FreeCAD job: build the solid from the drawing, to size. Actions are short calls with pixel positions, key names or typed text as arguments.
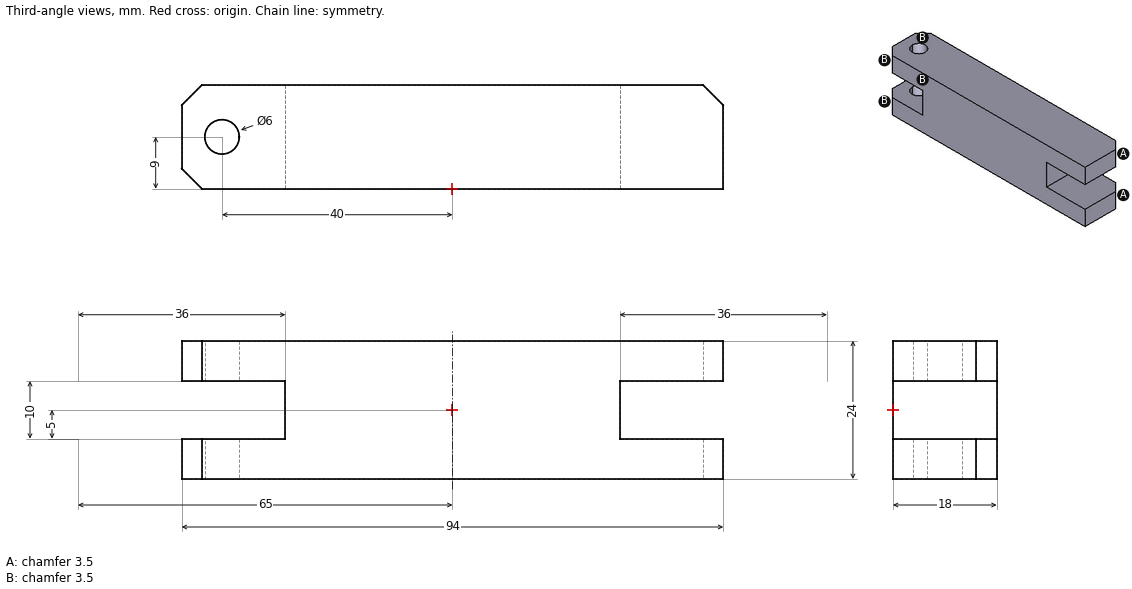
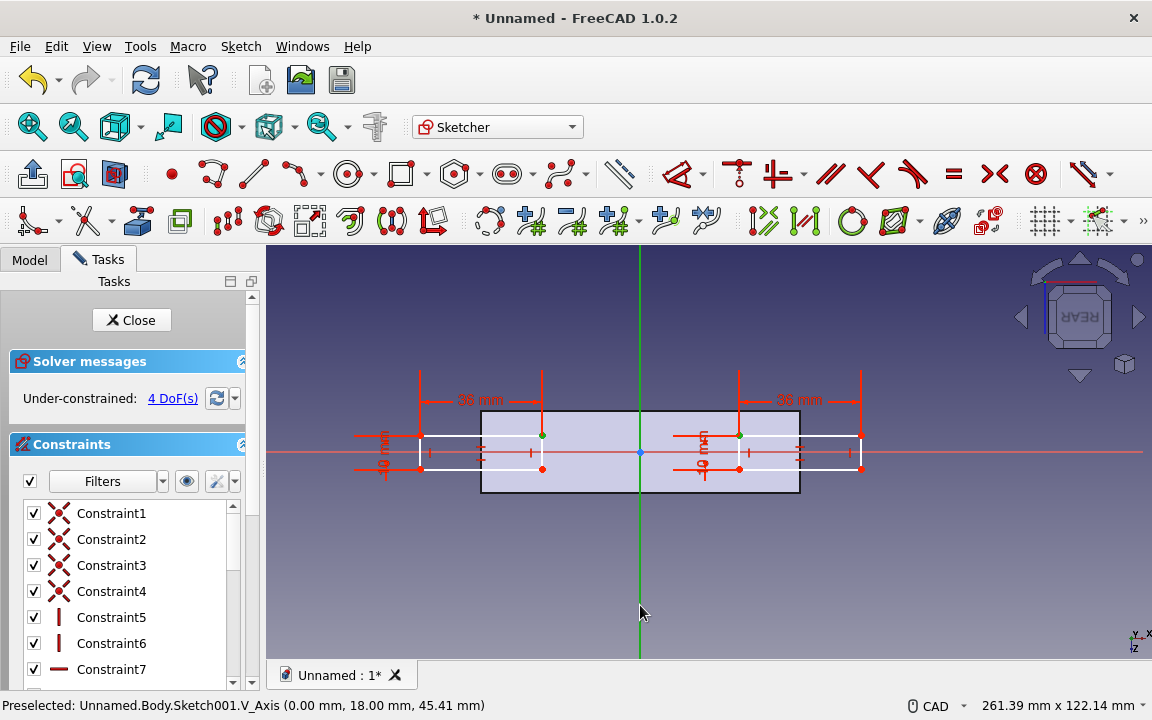
key(s)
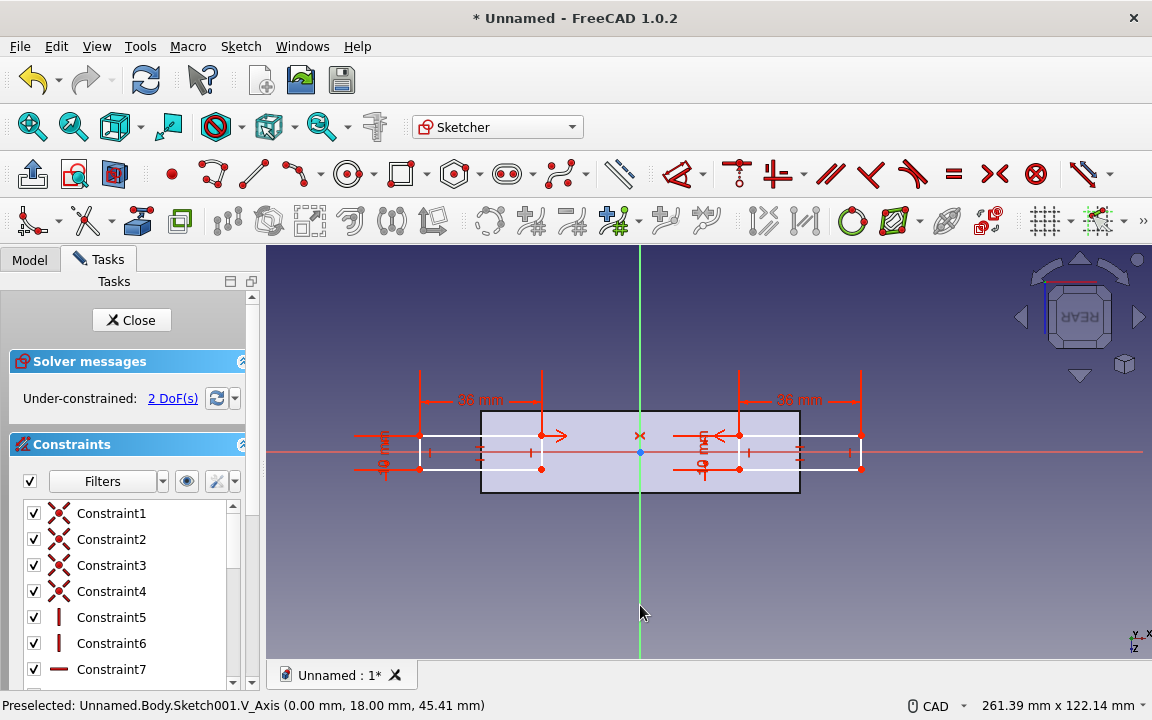
key(d)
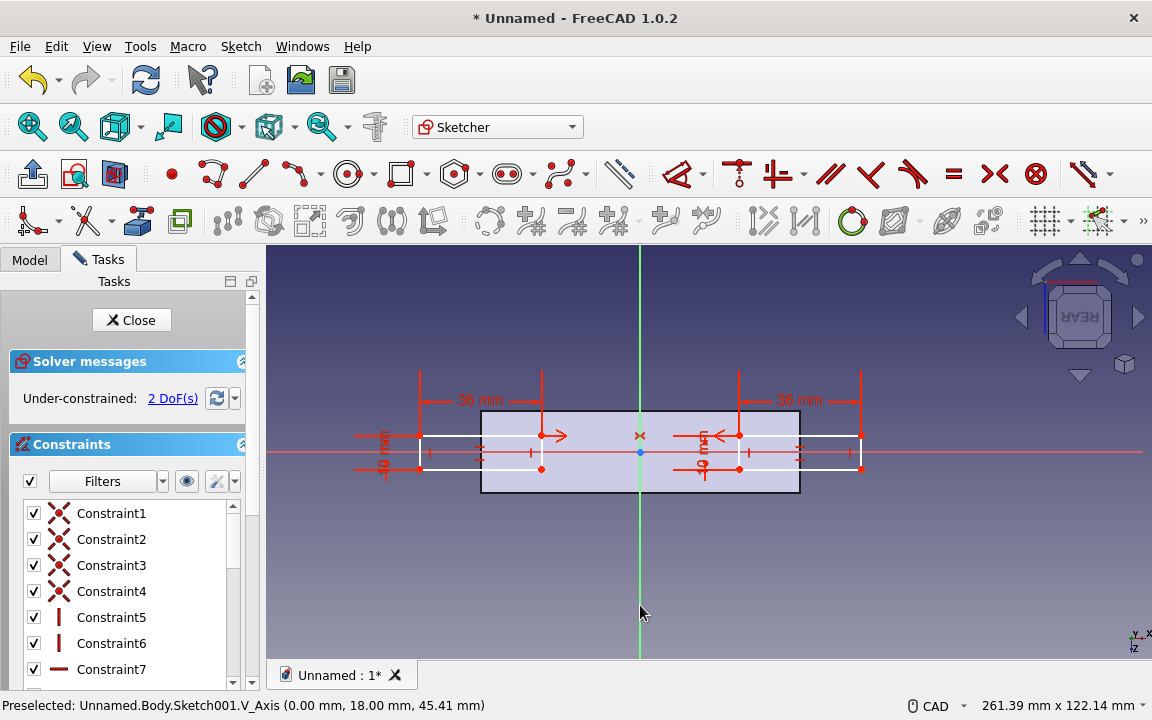
scroll(420, 436, up, 5)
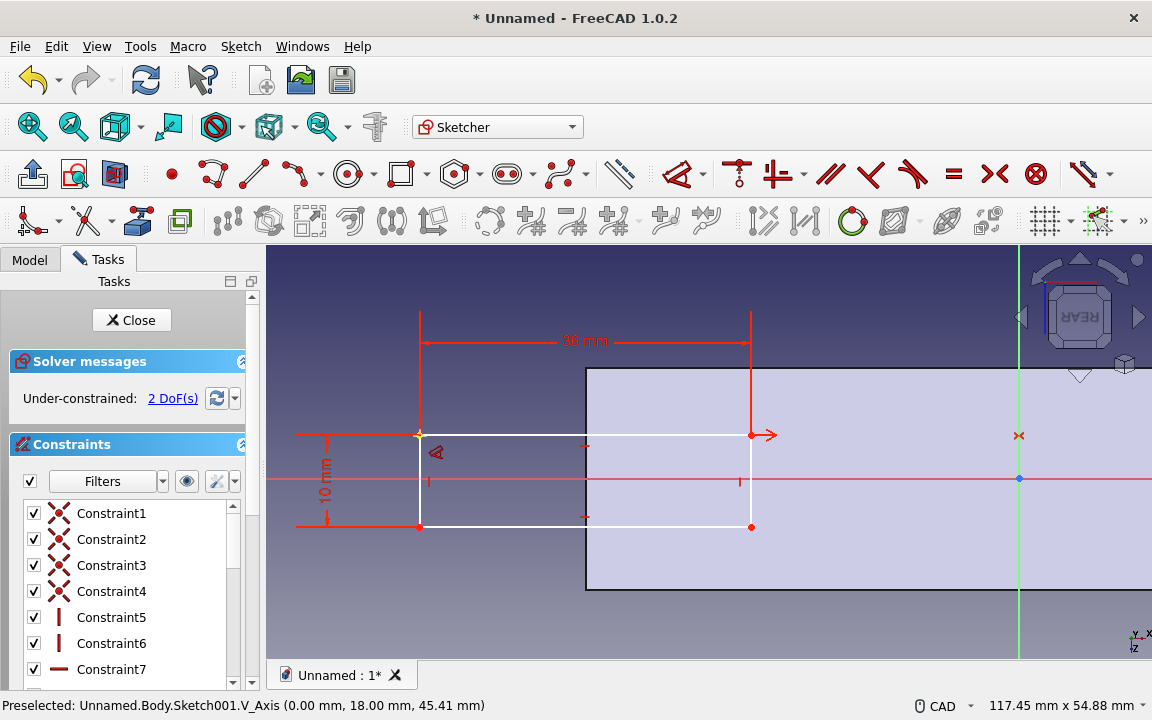
click(420, 435)
click(386, 457)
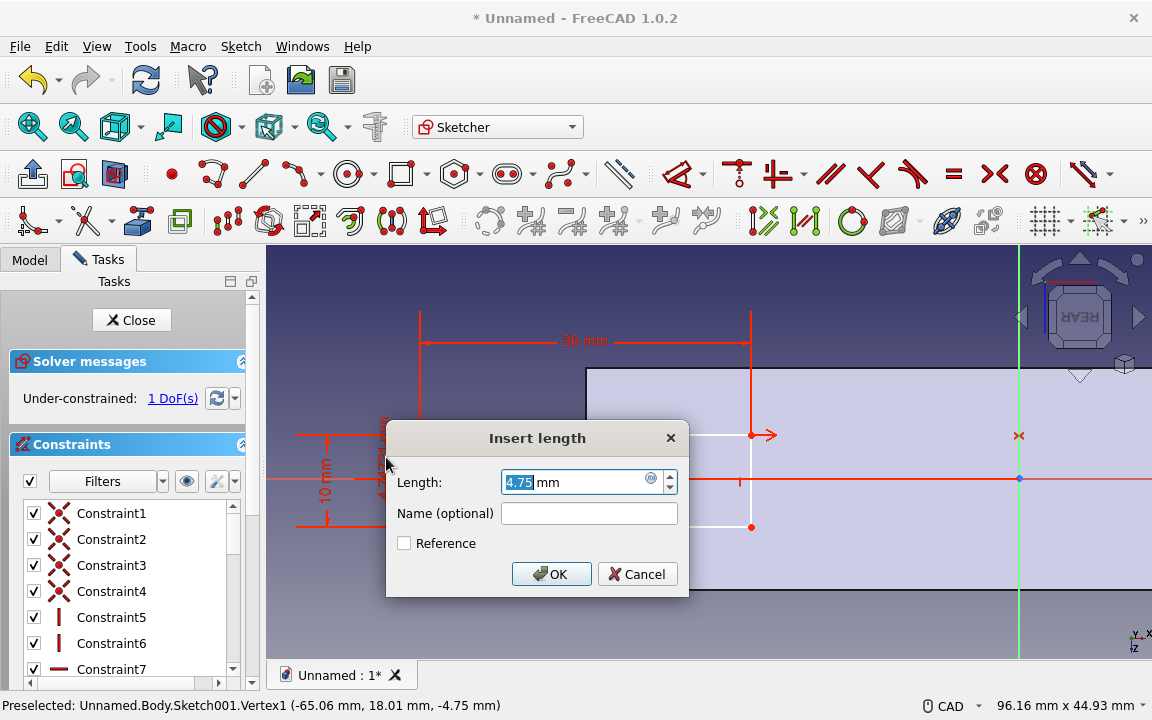
text(5)
key(Return)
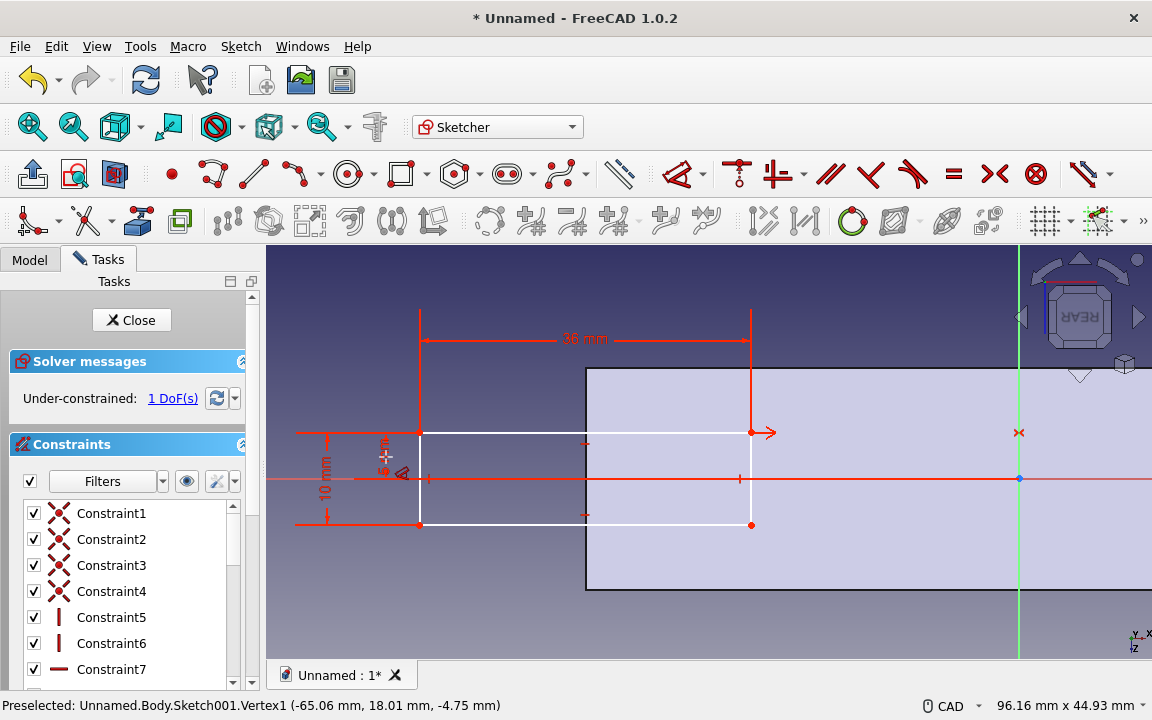
click(420, 433)
click(703, 399)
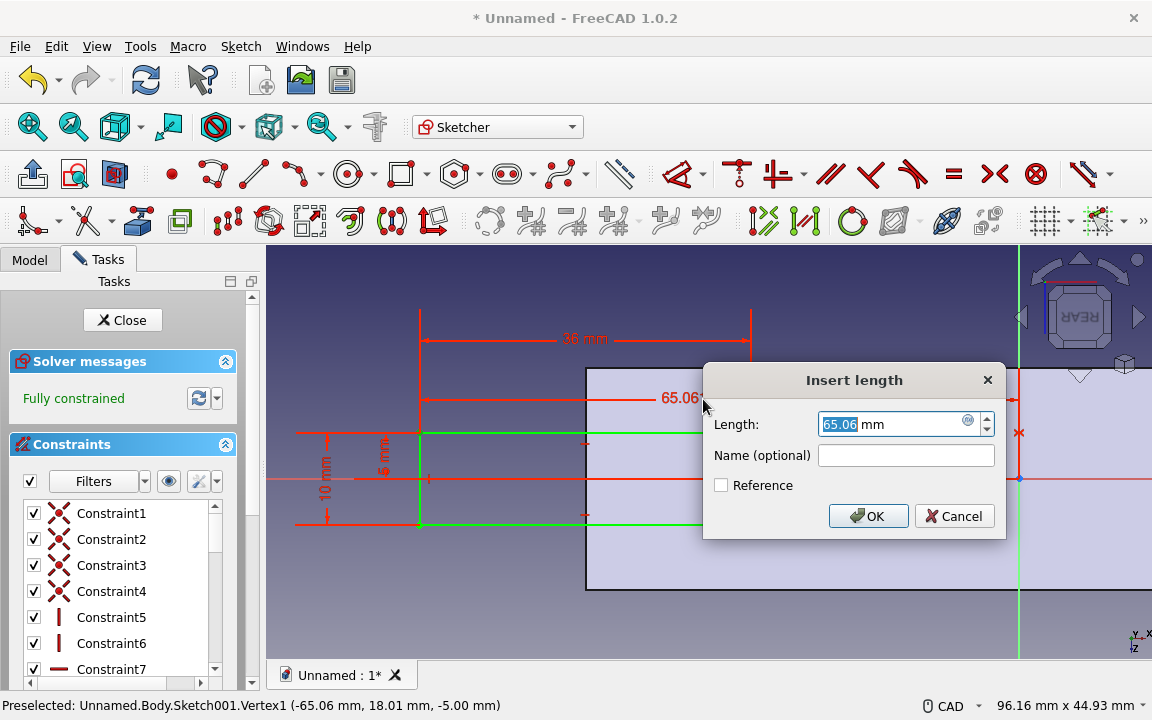
text(65)
key(Return)
key(Escape)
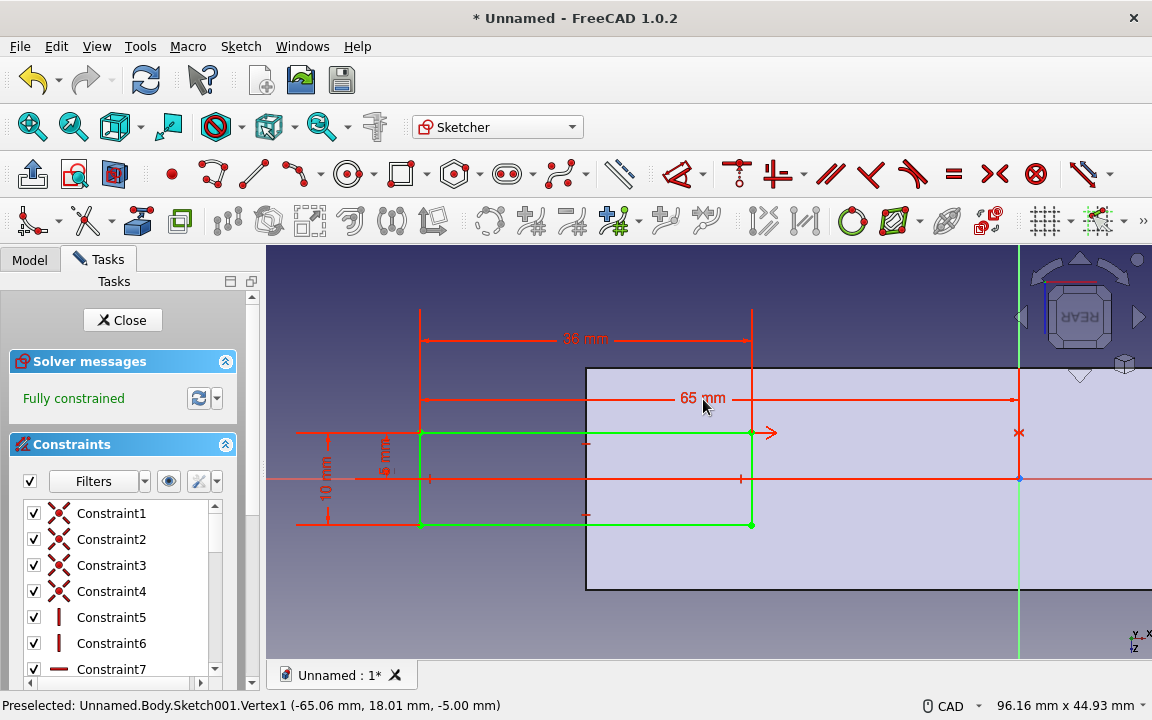
click(123, 320)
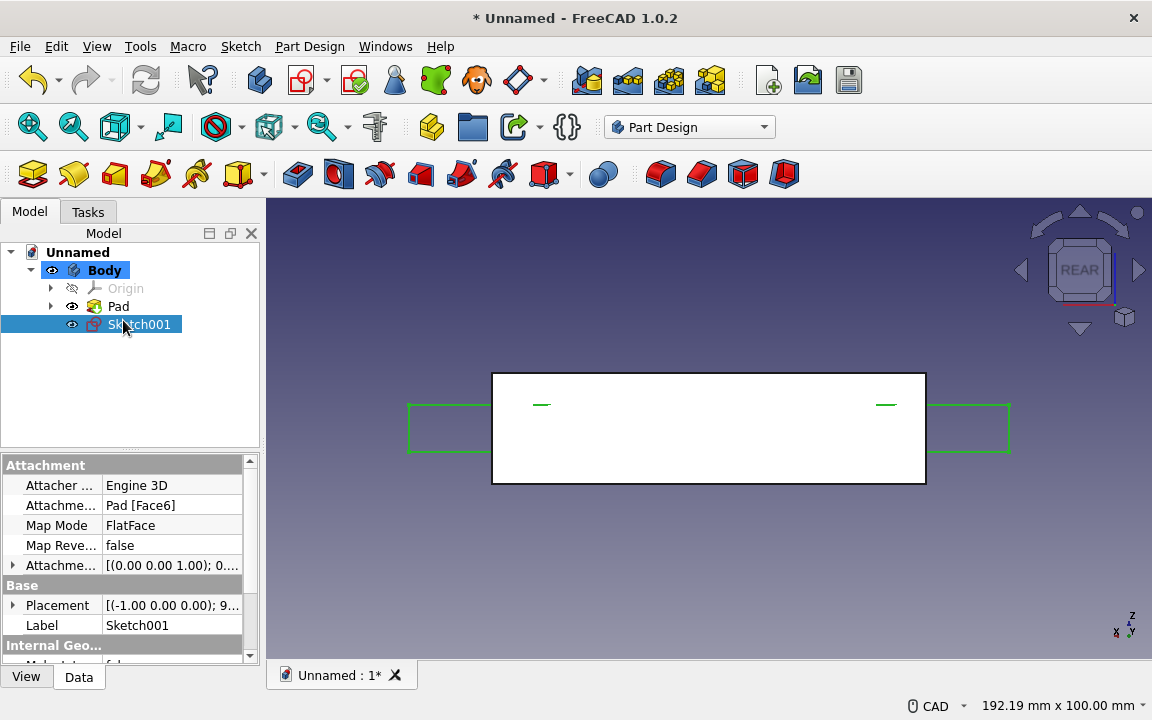
click(298, 174)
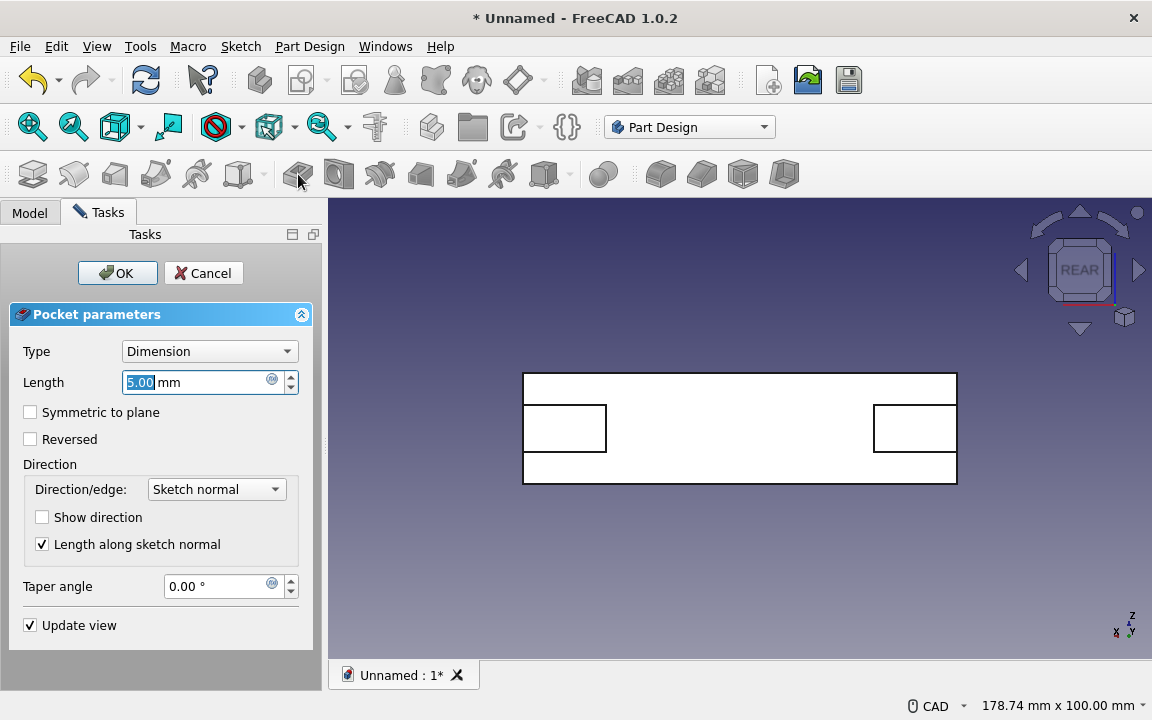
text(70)
key(Tab)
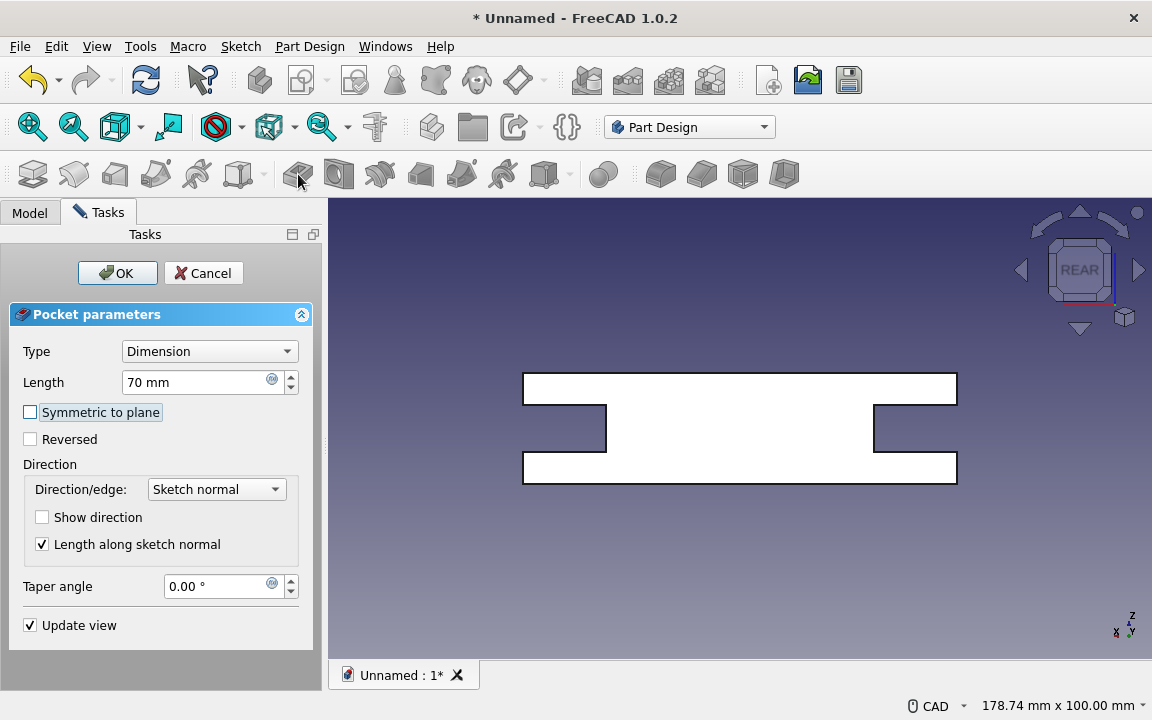
click(118, 273)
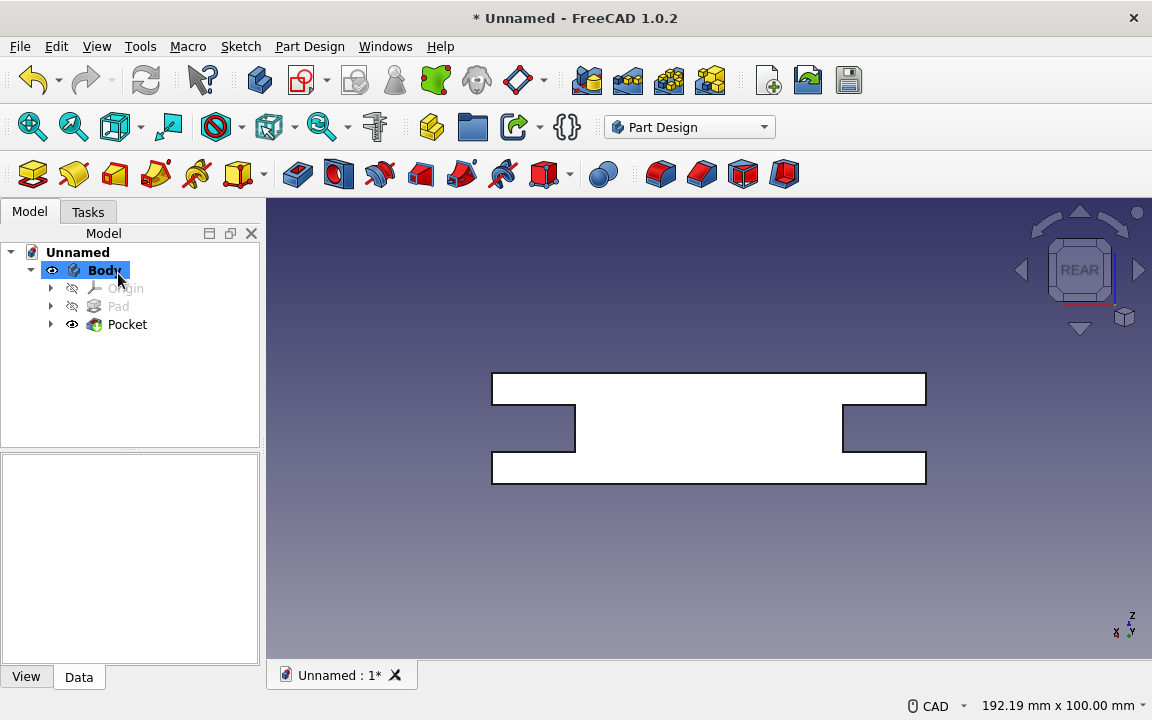
key(0)